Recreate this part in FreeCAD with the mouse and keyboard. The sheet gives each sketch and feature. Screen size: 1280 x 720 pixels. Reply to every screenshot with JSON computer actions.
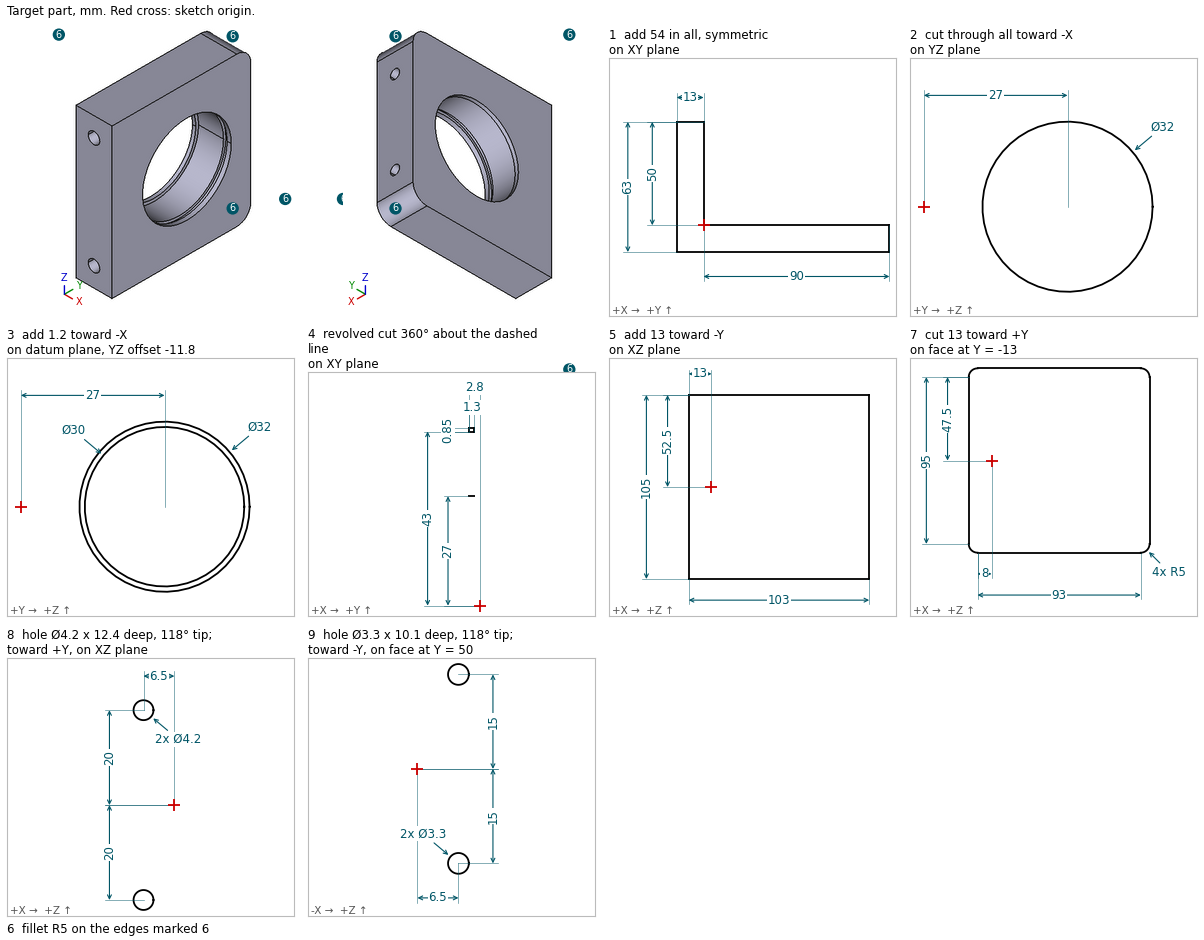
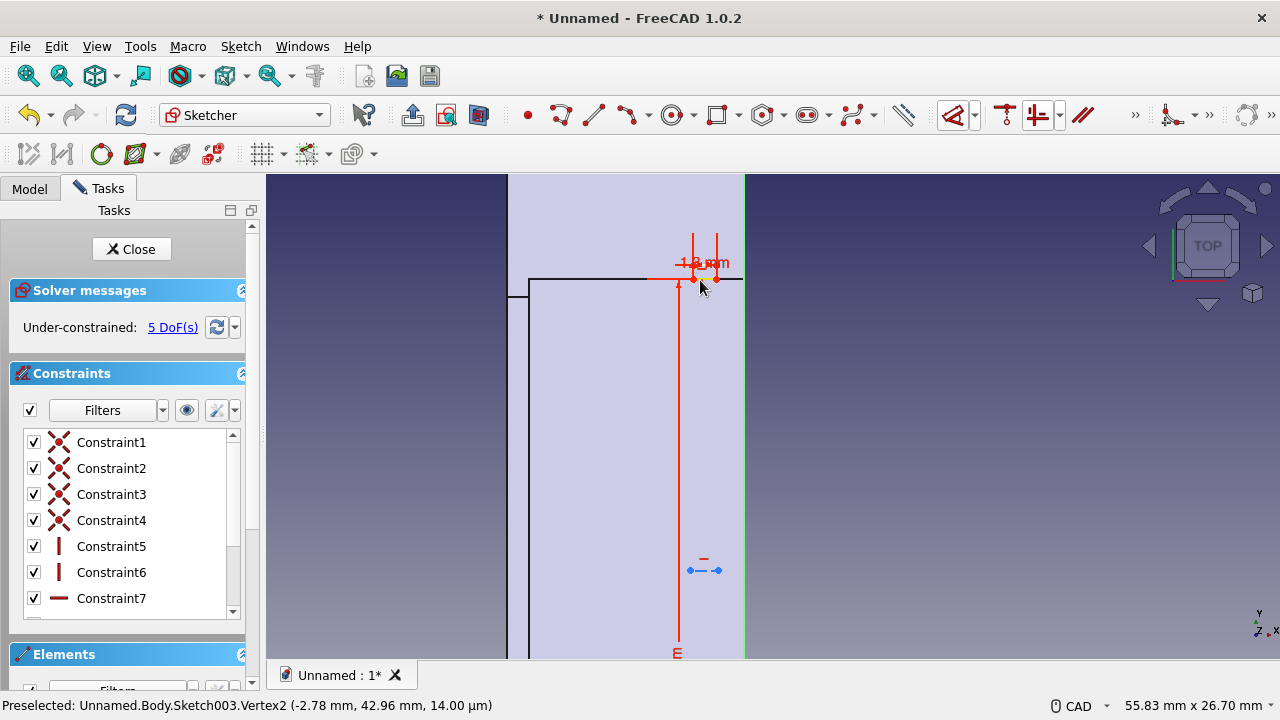
{"action": "left_click", "coordinate": [691, 571]}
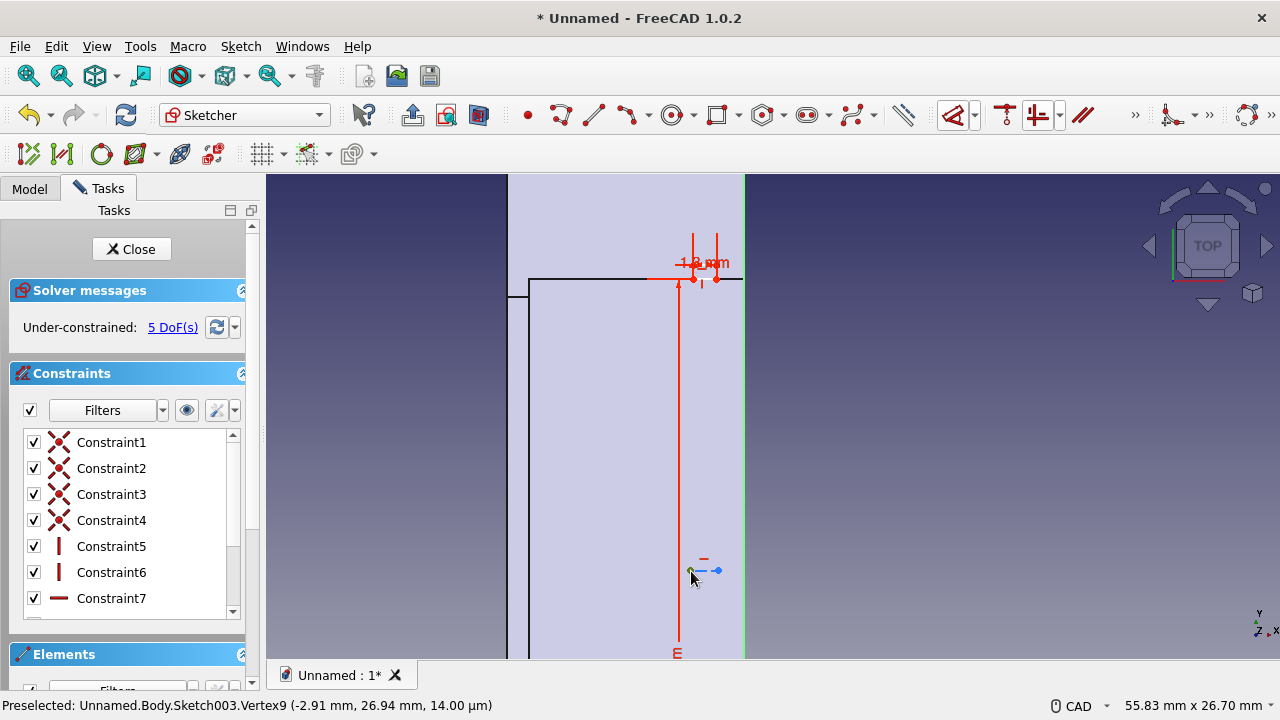
{"action": "key", "text": "i"}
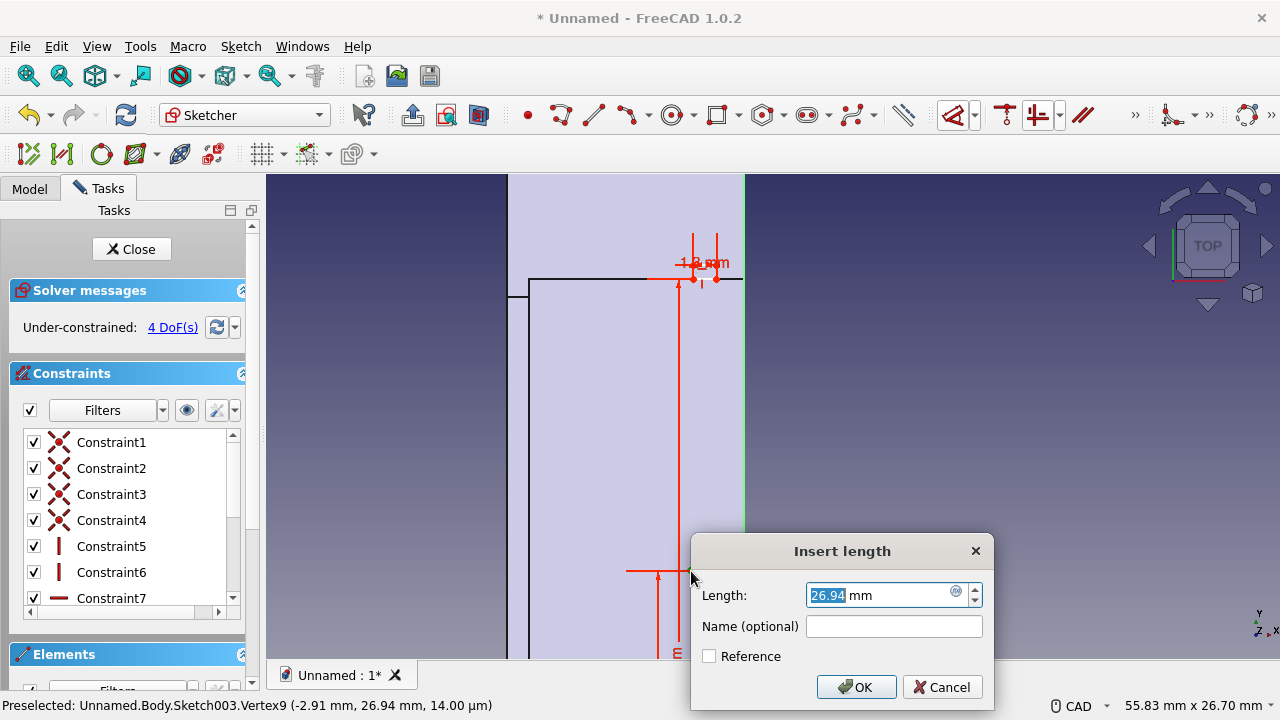
{"action": "type", "text": "27"}
{"action": "key", "text": "Return"}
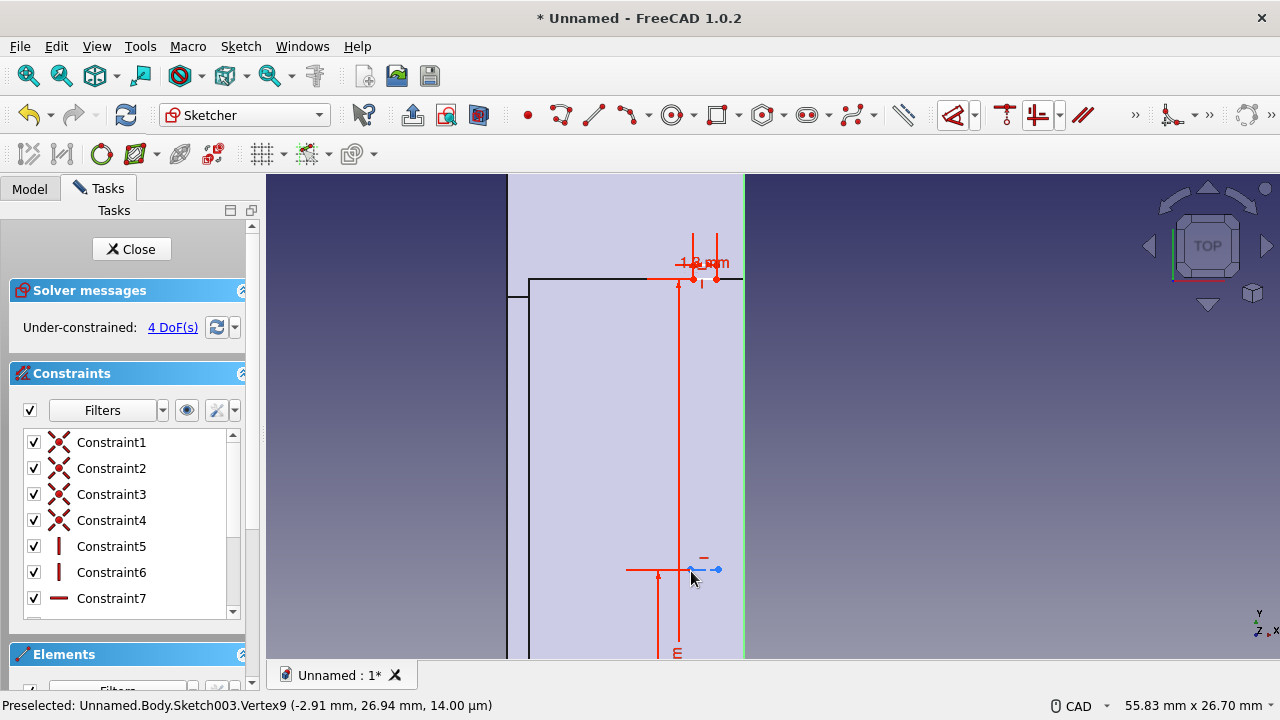
{"action": "scroll", "coordinate": [693, 272], "scroll_direction": "up", "scroll_amount": 5}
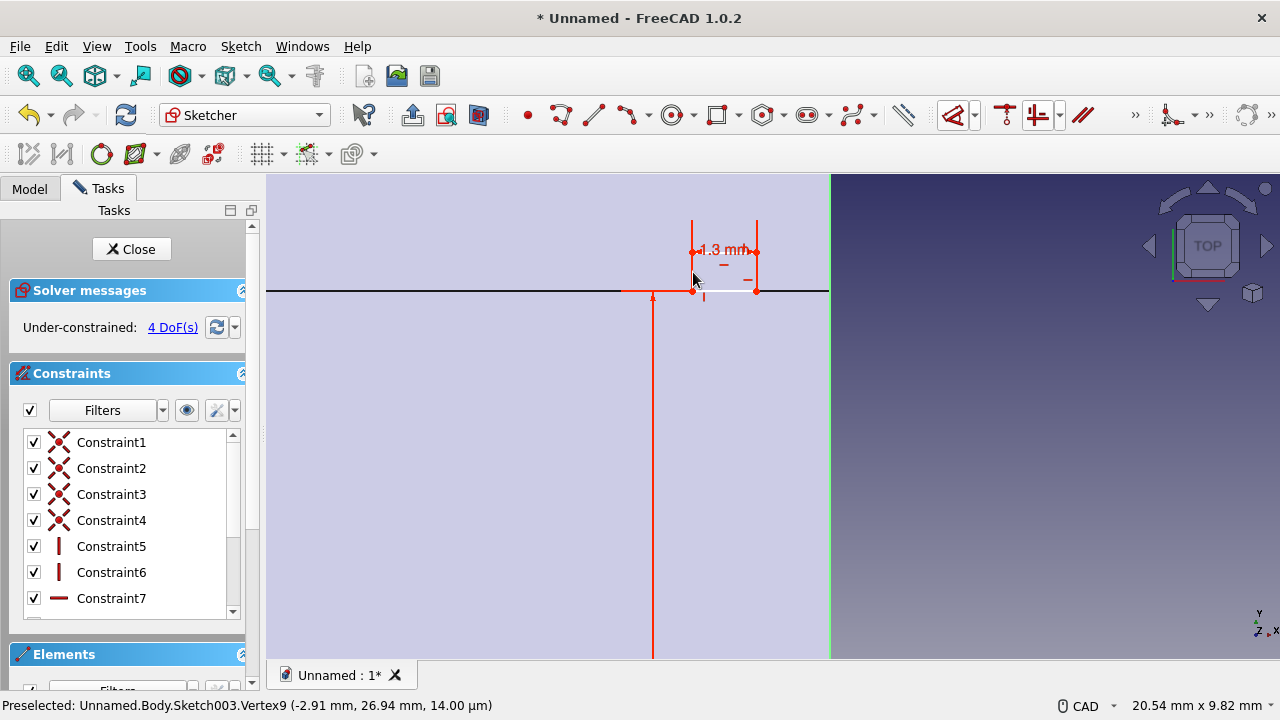
{"action": "left_click", "coordinate": [692, 272]}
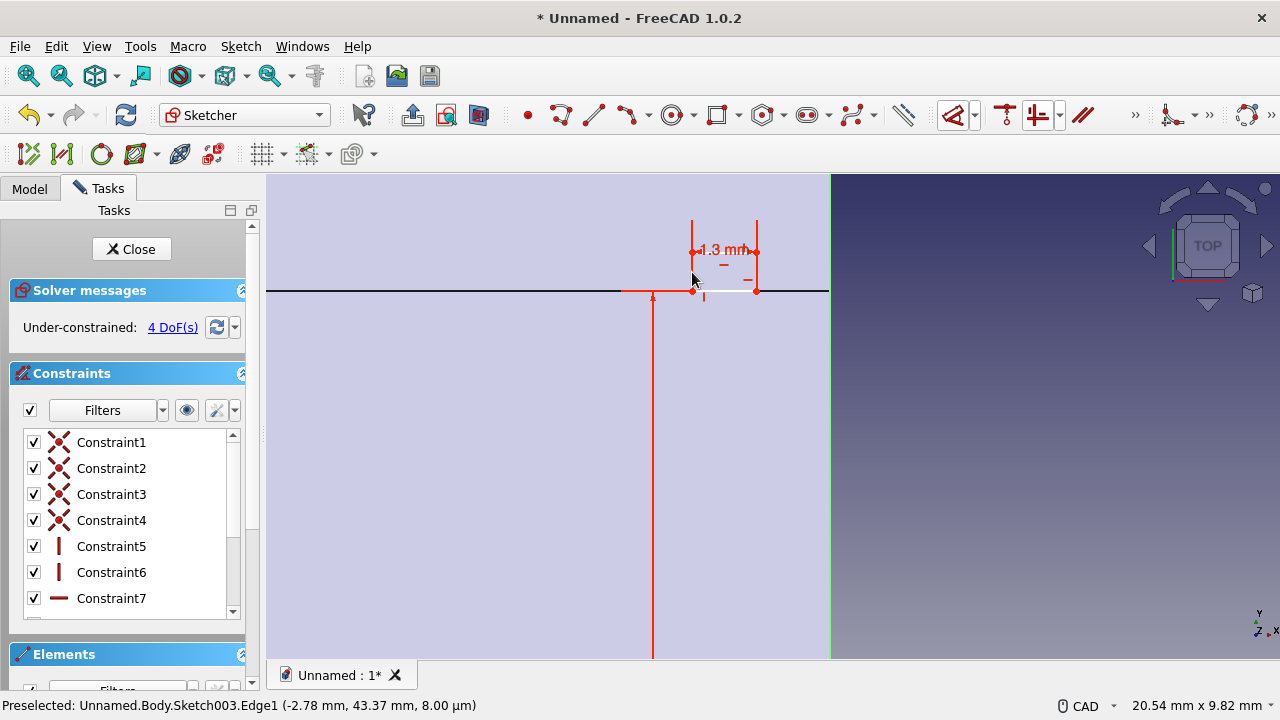
{"action": "left_click", "coordinate": [974, 116]}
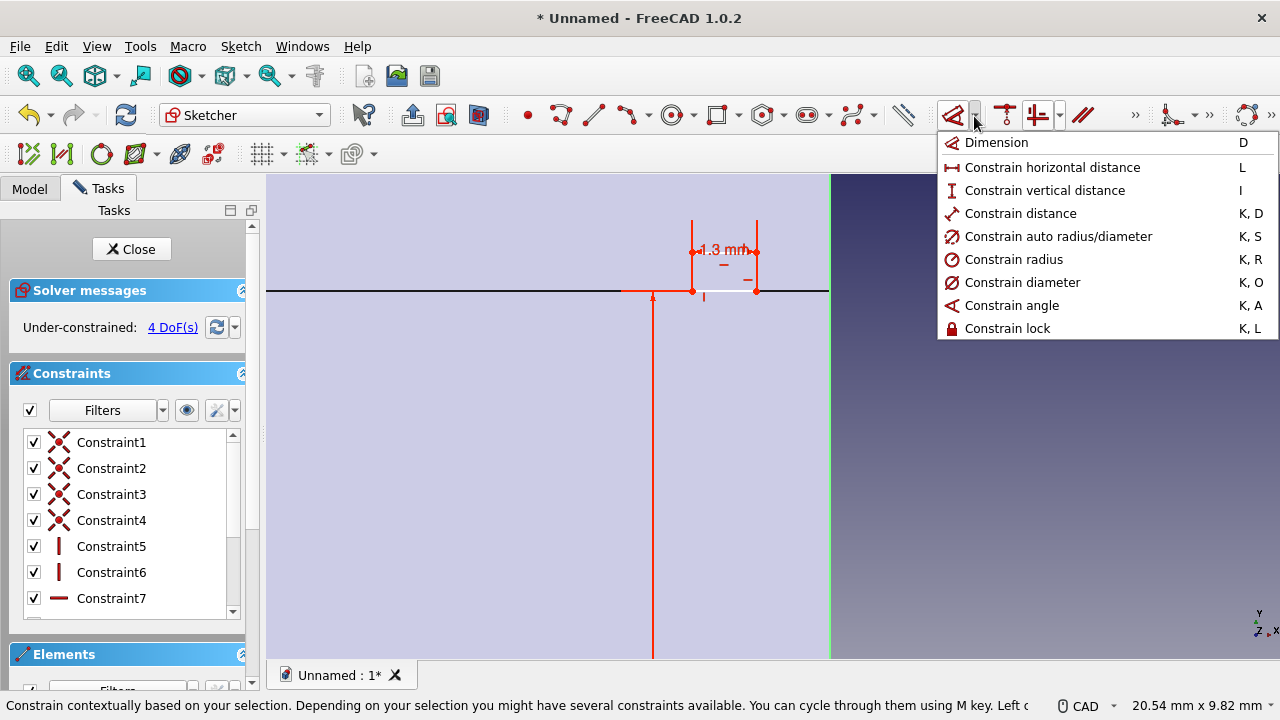
{"action": "left_click", "coordinate": [1108, 190]}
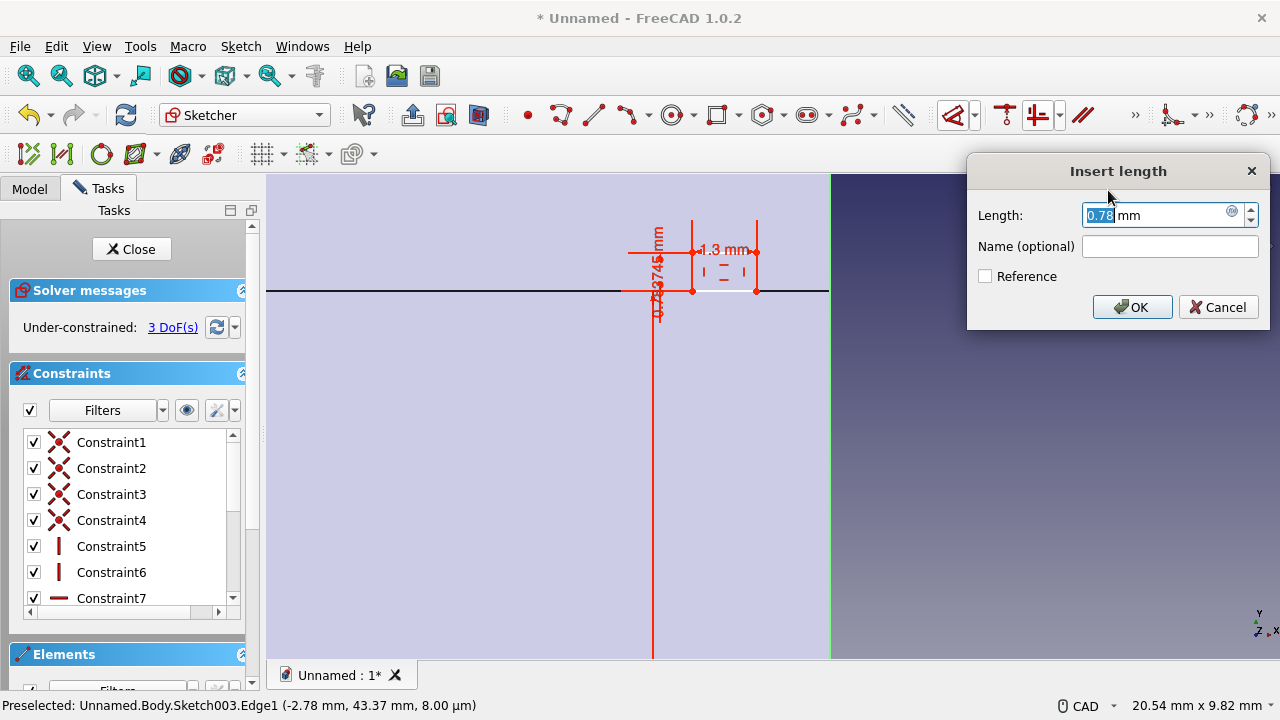
{"action": "type", "text": "0.85"}
{"action": "key", "text": "Return"}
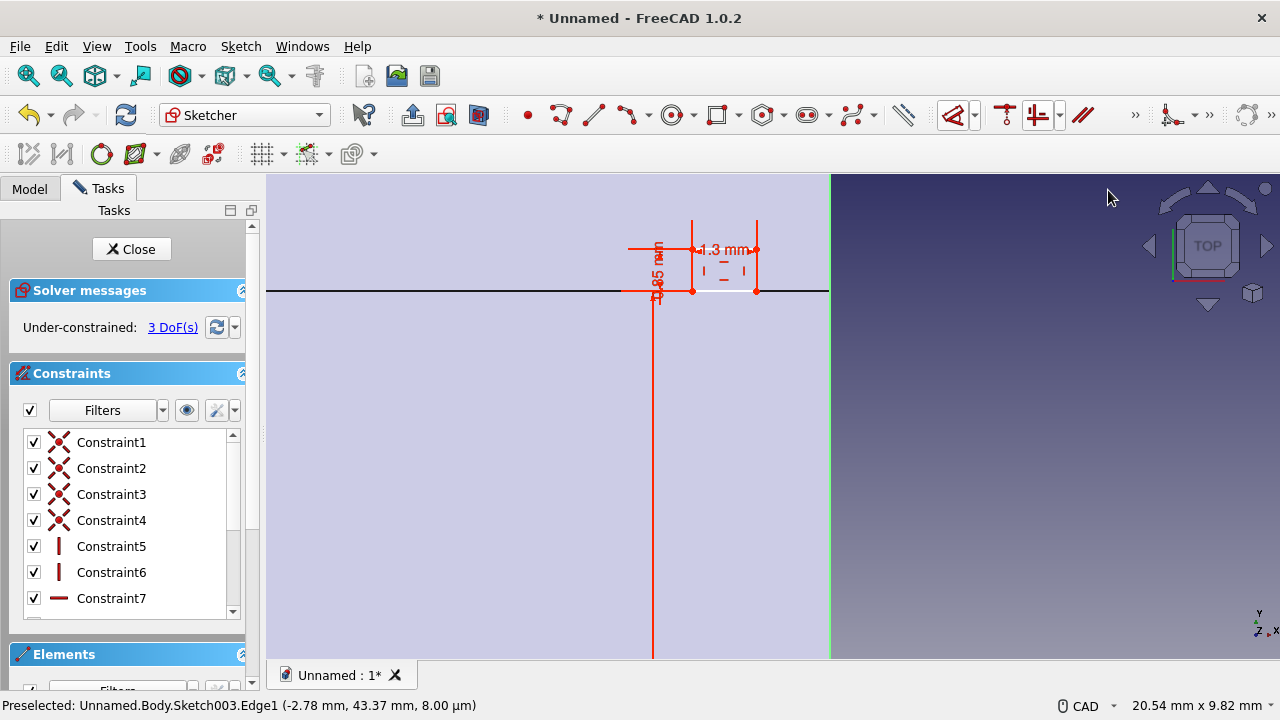
{"action": "left_click", "coordinate": [692, 249]}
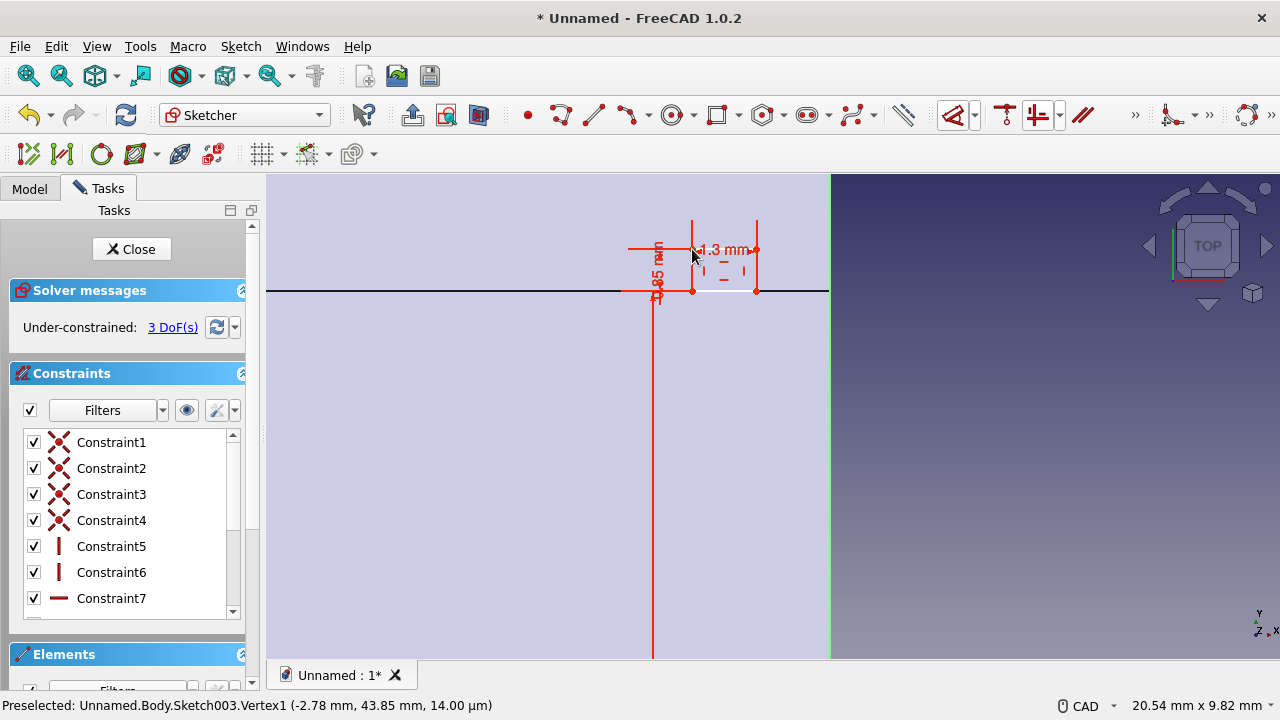
{"action": "key", "text": "l"}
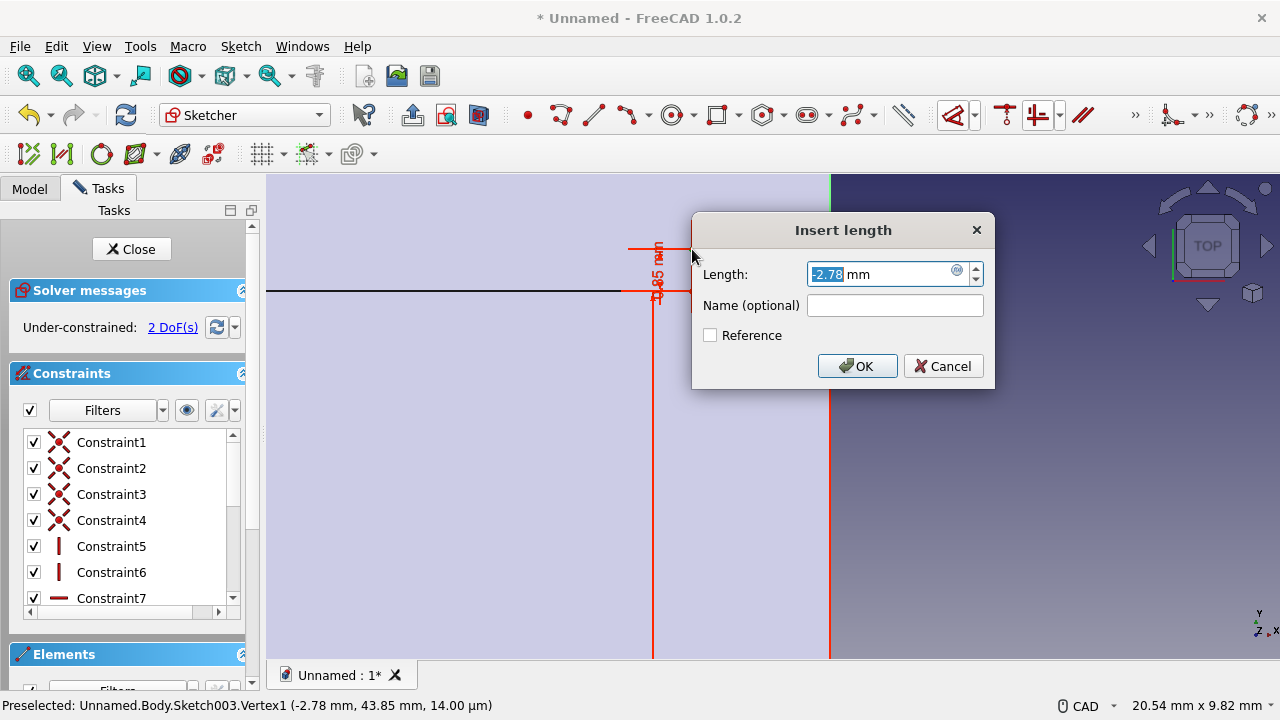
{"action": "type", "text": "-2.8"}
{"action": "key", "text": "Return"}